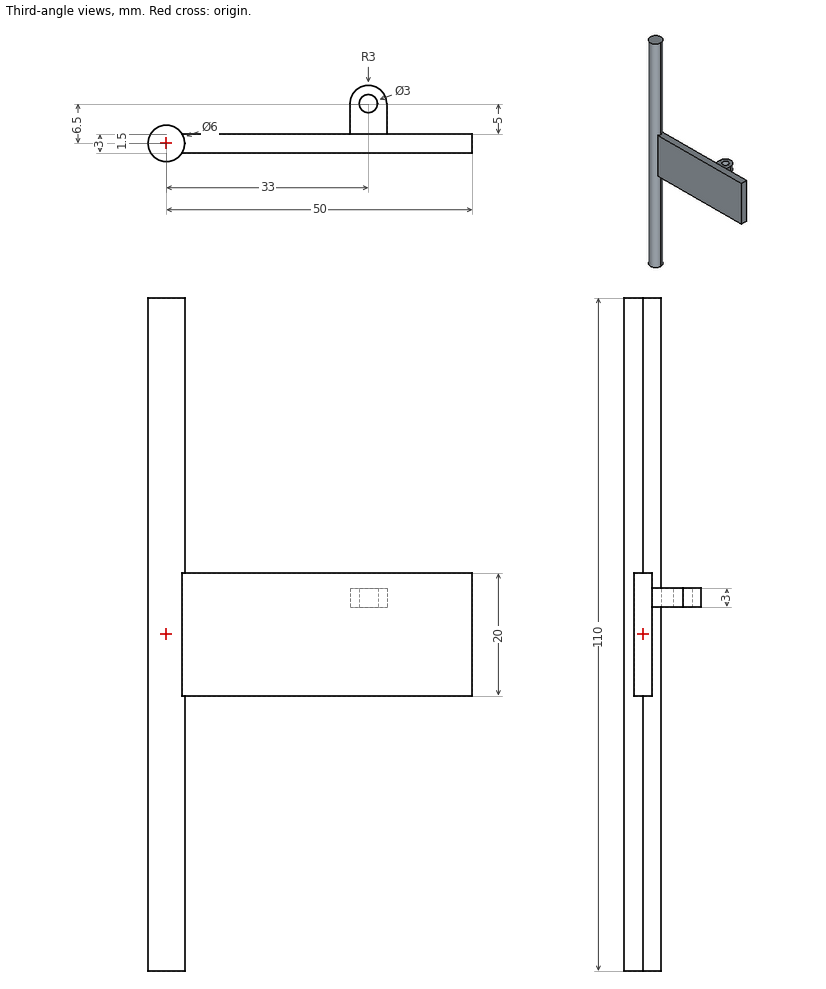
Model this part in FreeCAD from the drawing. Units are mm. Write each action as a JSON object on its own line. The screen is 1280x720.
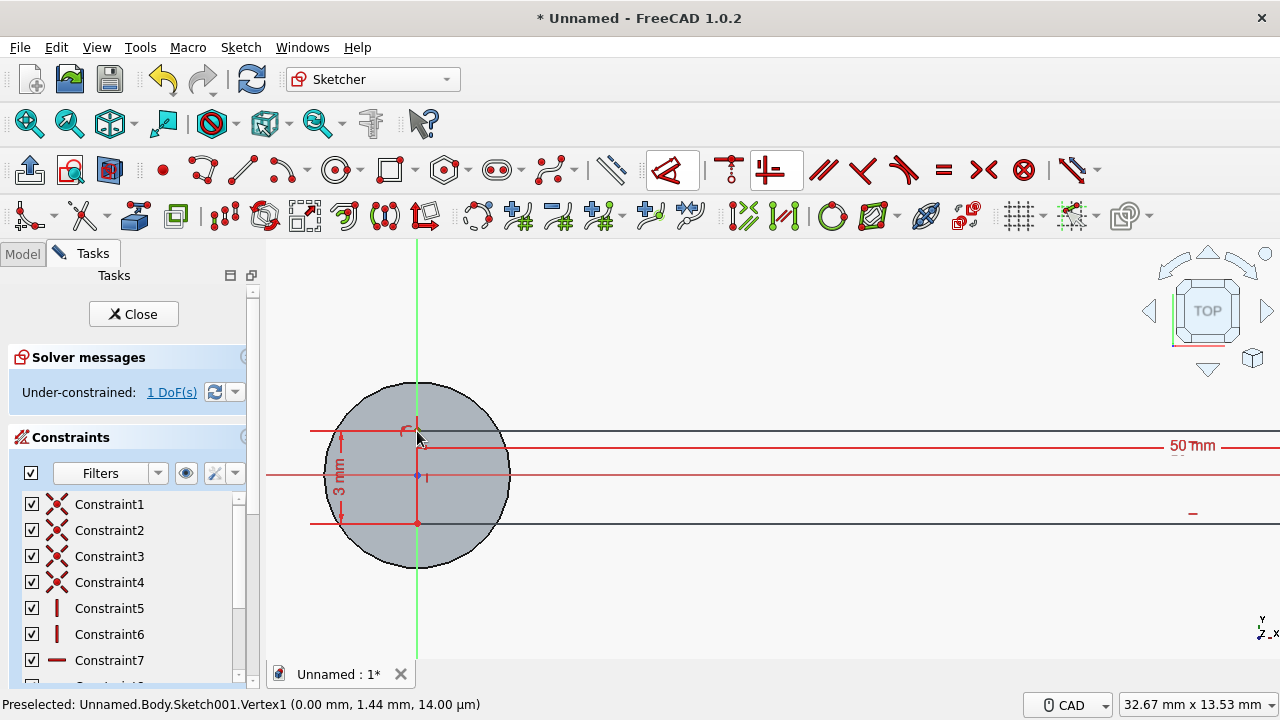
{"action": "key", "text": "i"}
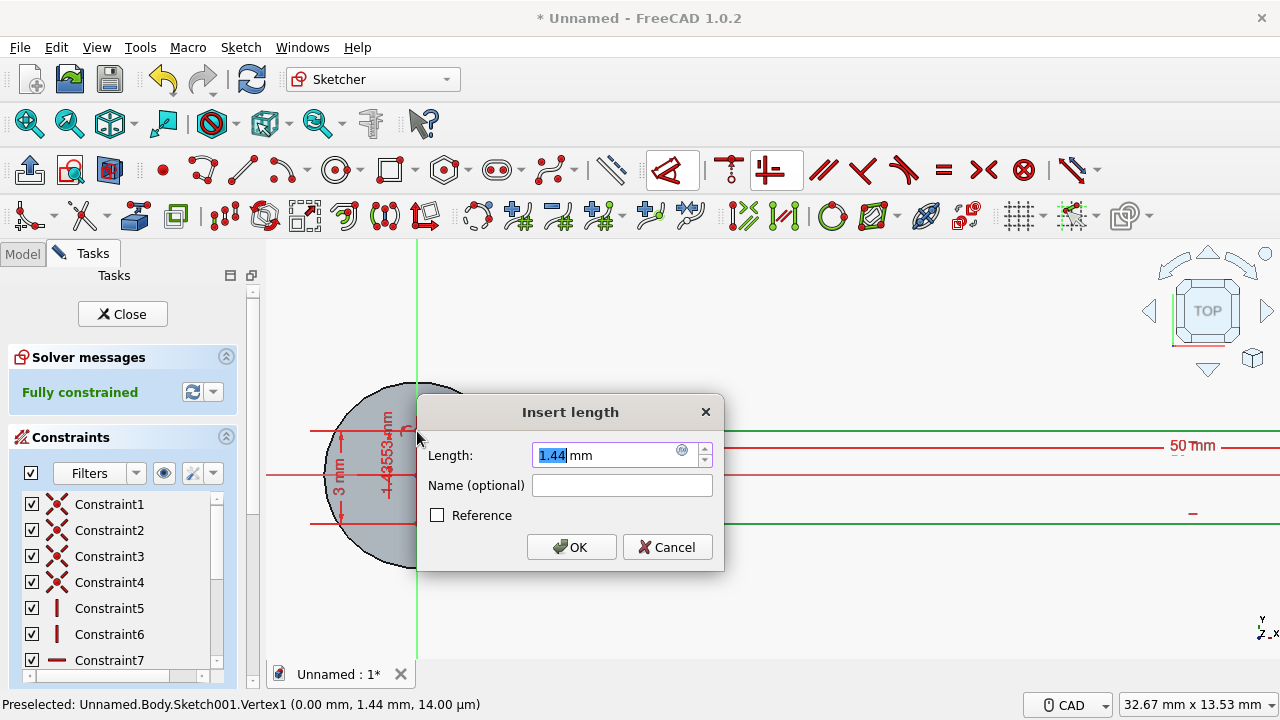
{"action": "type", "text": "1.5"}
{"action": "key", "text": "Return"}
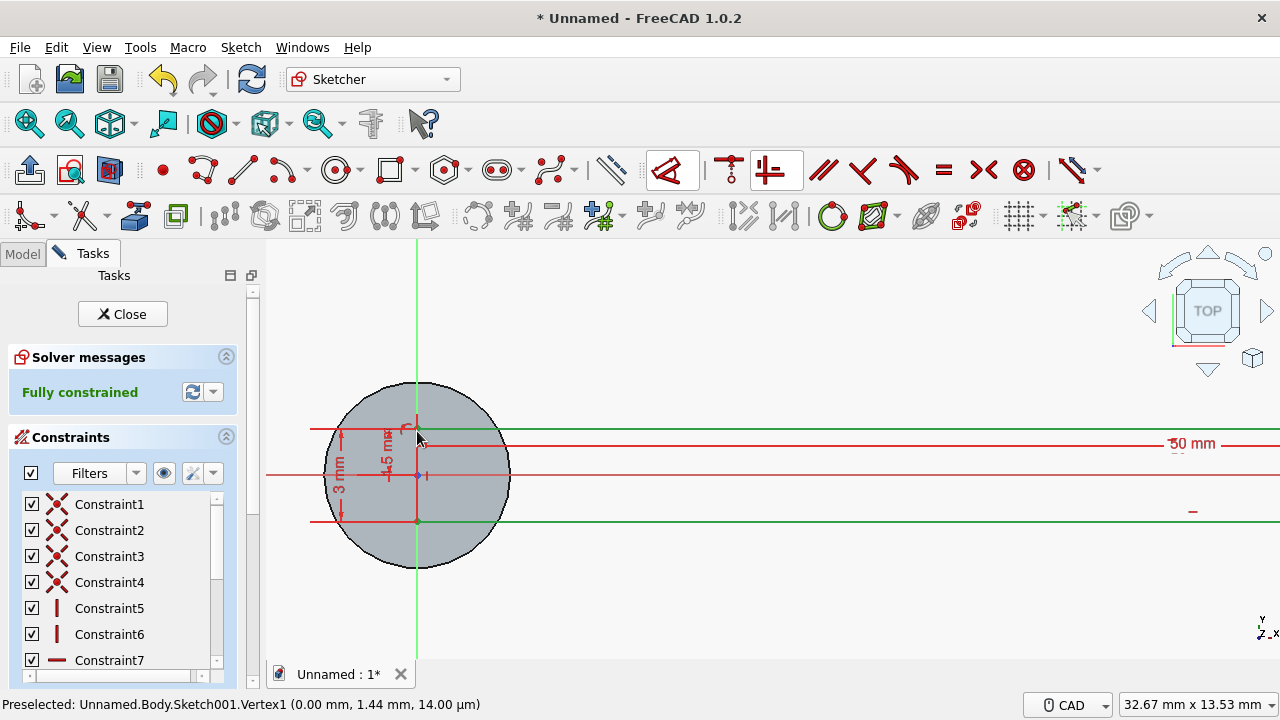
{"action": "left_click", "coordinate": [123, 314]}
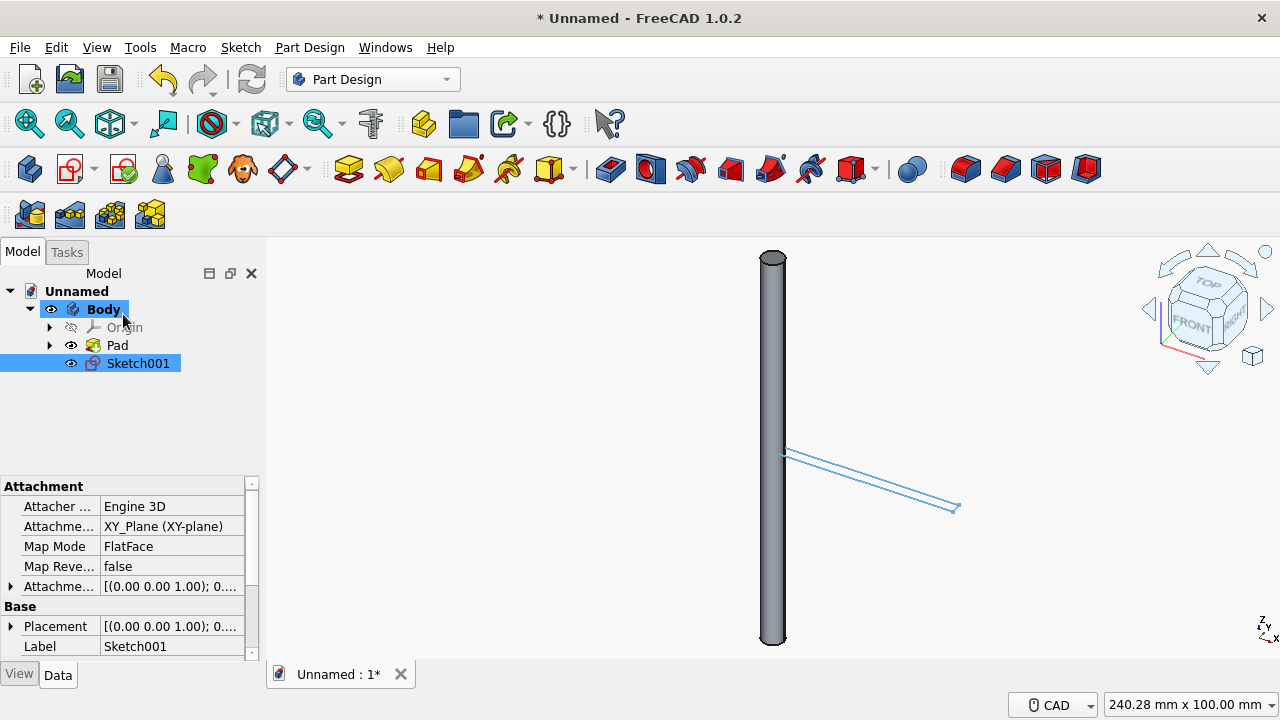
{"action": "left_click", "coordinate": [350, 170]}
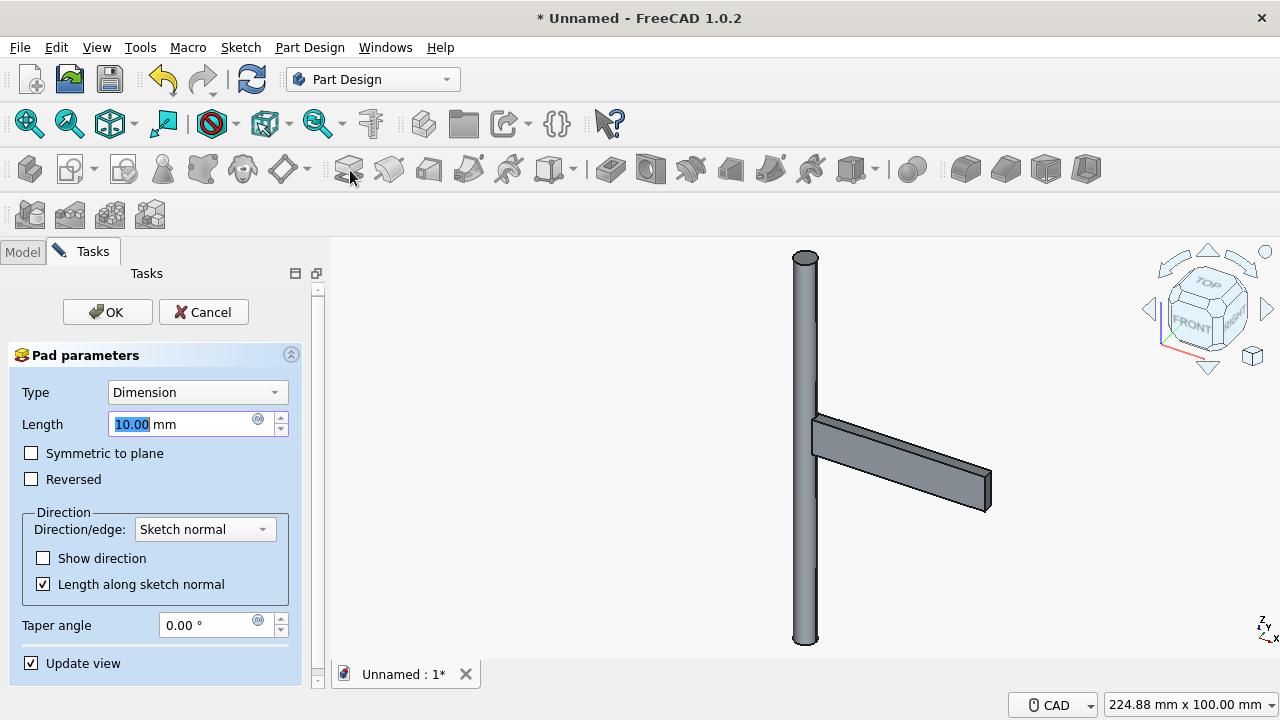
{"action": "type", "text": "20"}
{"action": "key", "text": "Tab"}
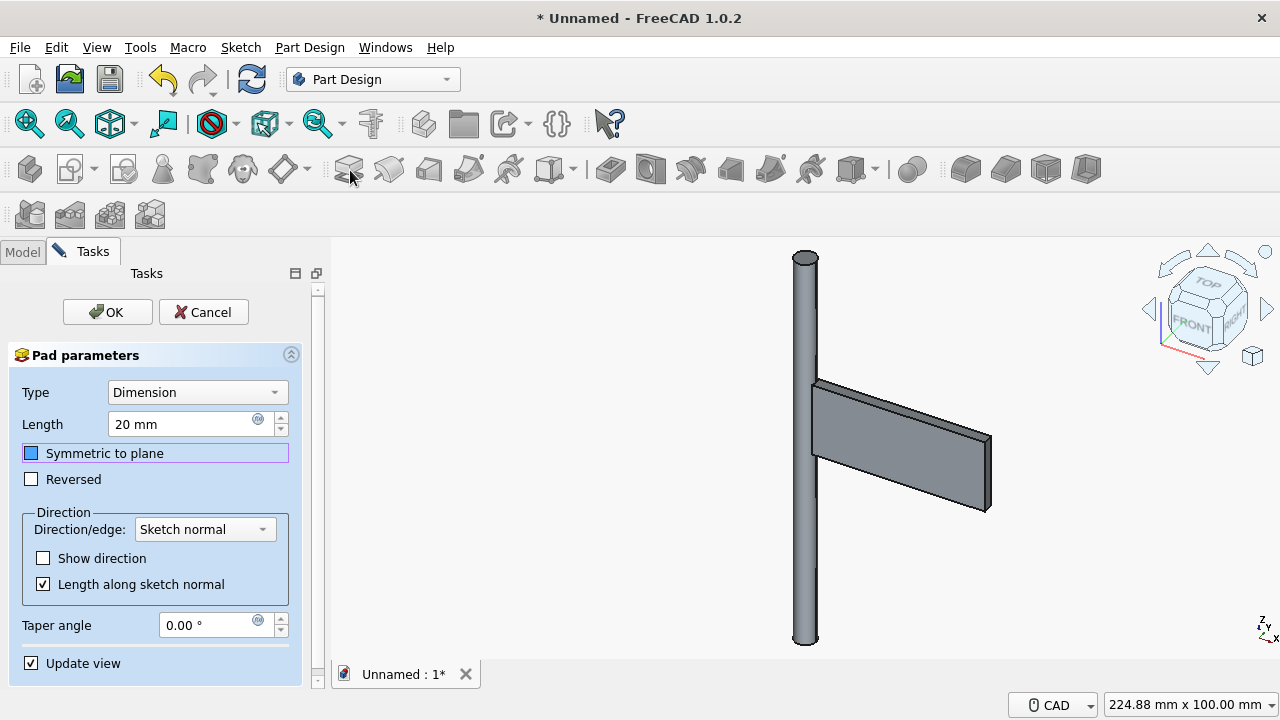
{"action": "left_click", "coordinate": [30, 453]}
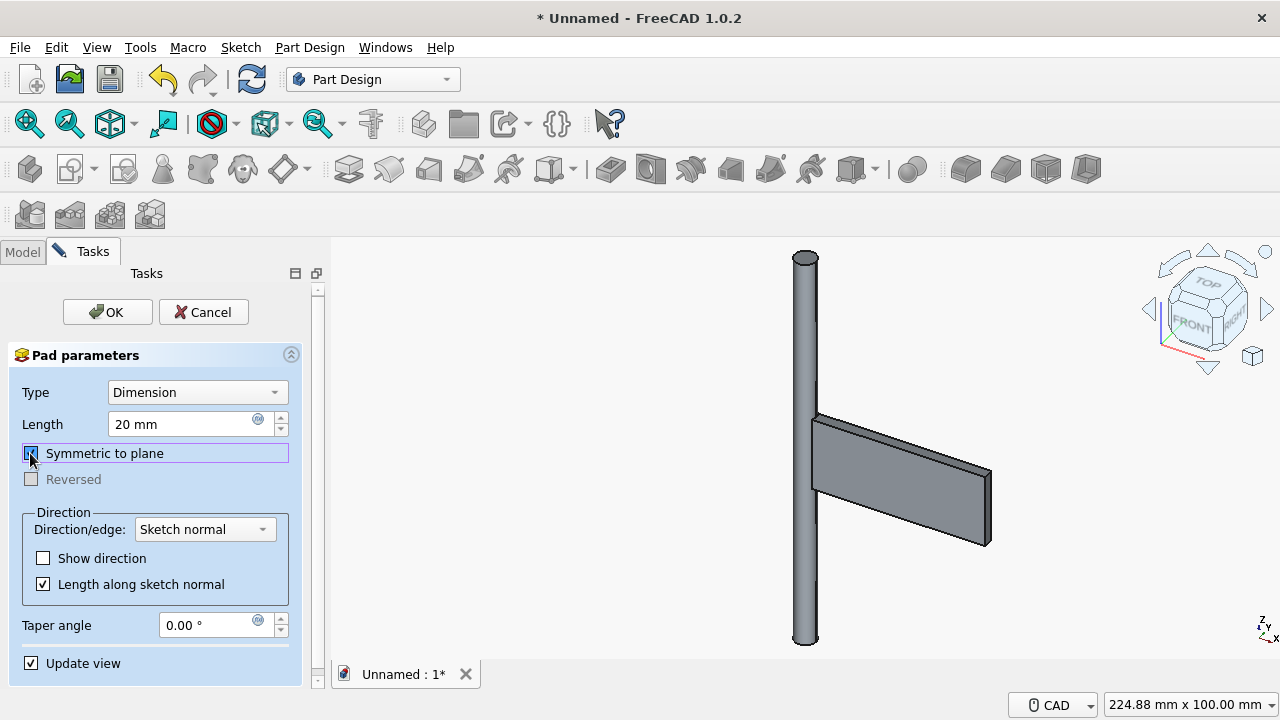
{"action": "left_click", "coordinate": [108, 312]}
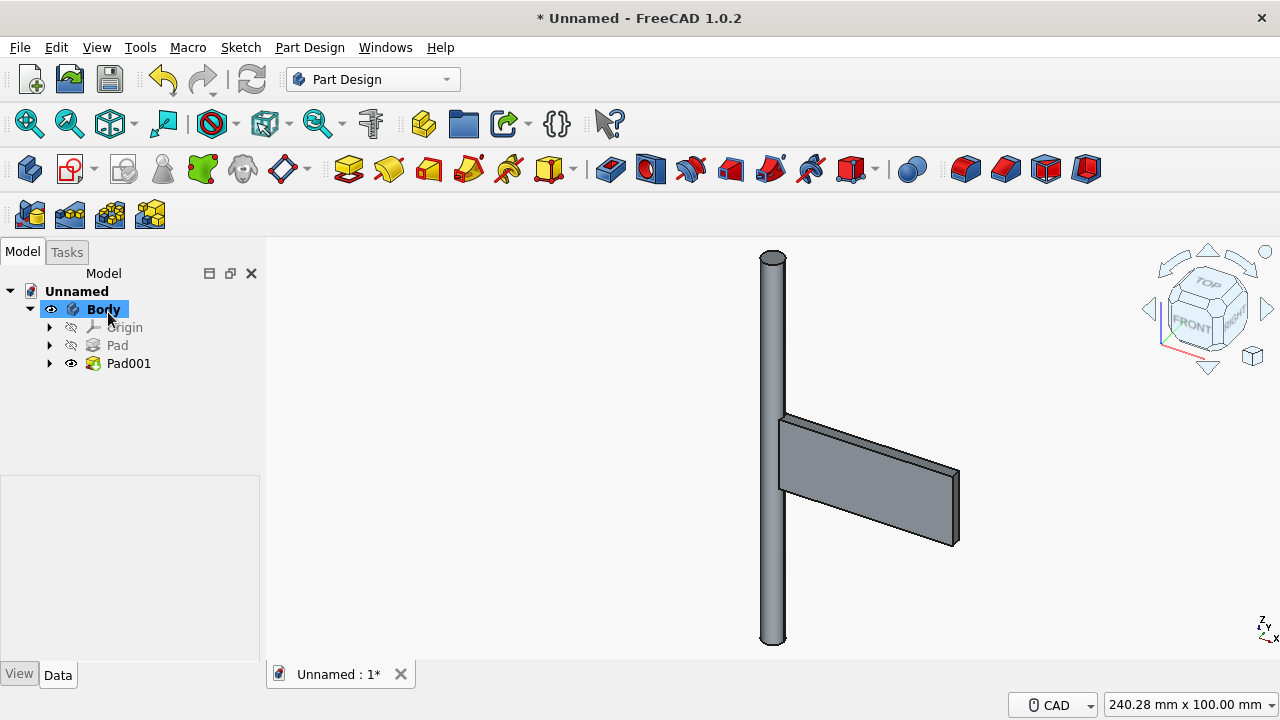
{"action": "left_click", "coordinate": [30, 124]}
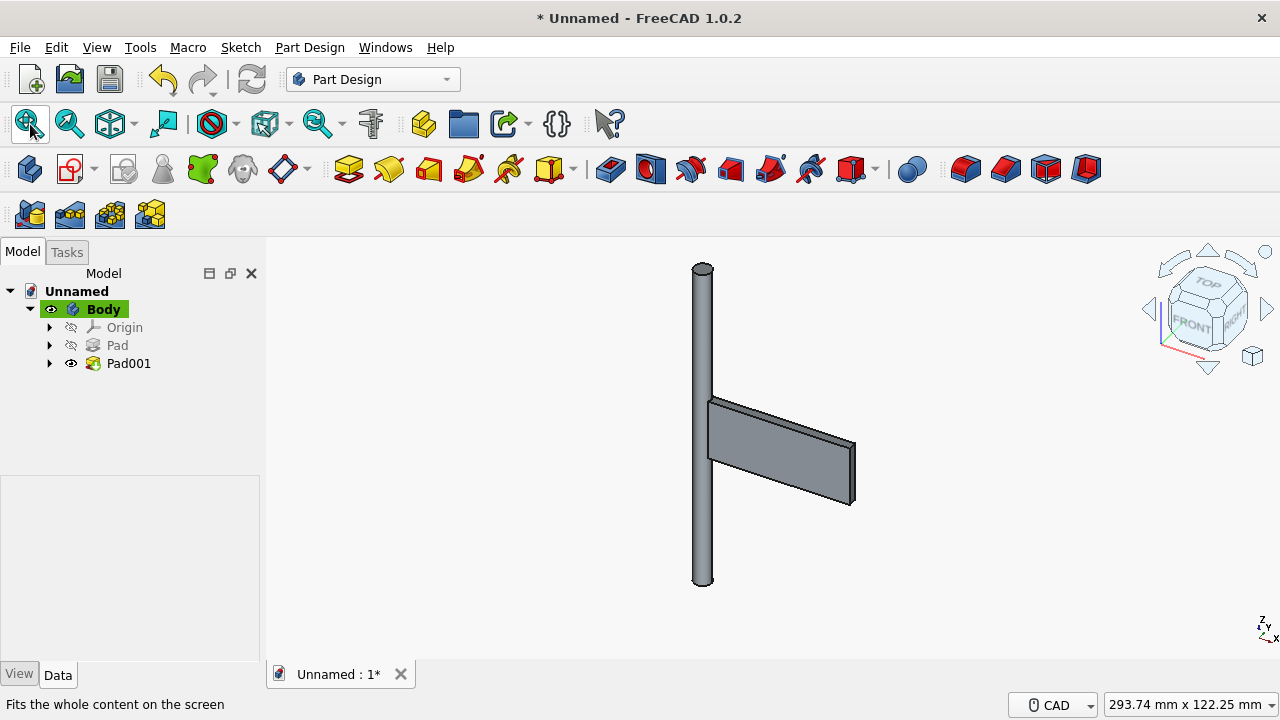
{"action": "left_click", "coordinate": [50, 327]}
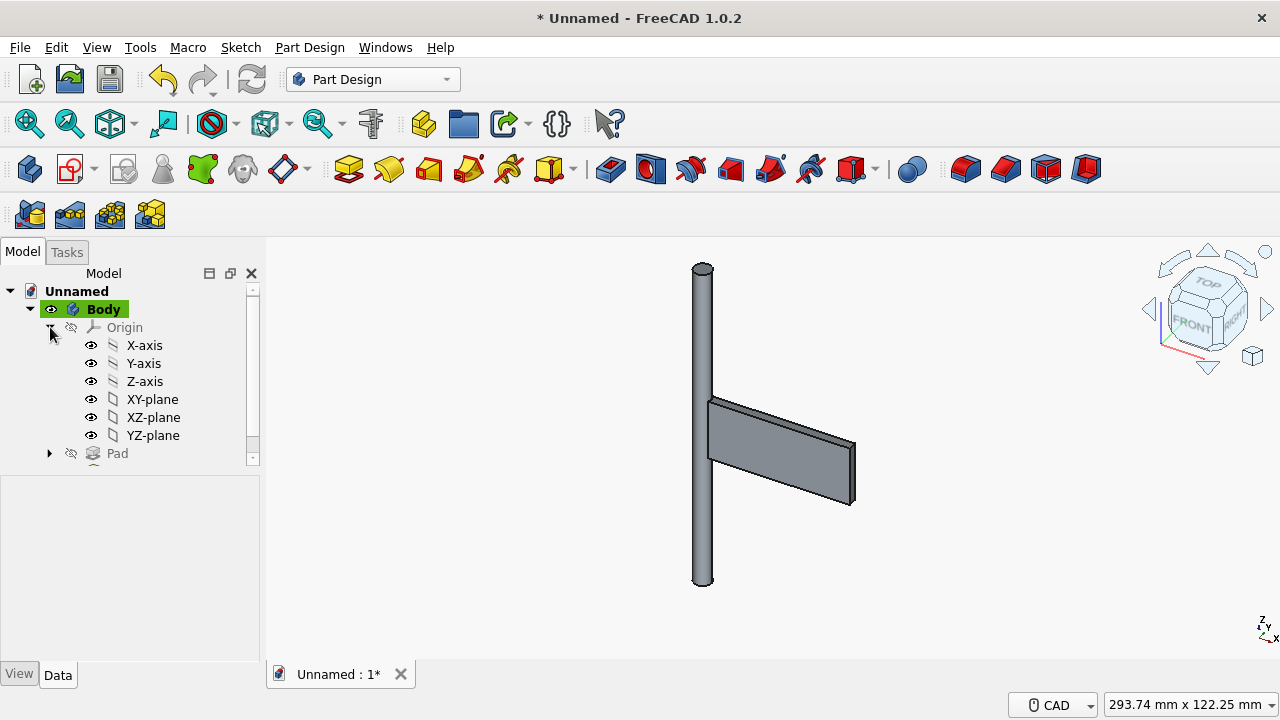
{"action": "left_click", "coordinate": [136, 399]}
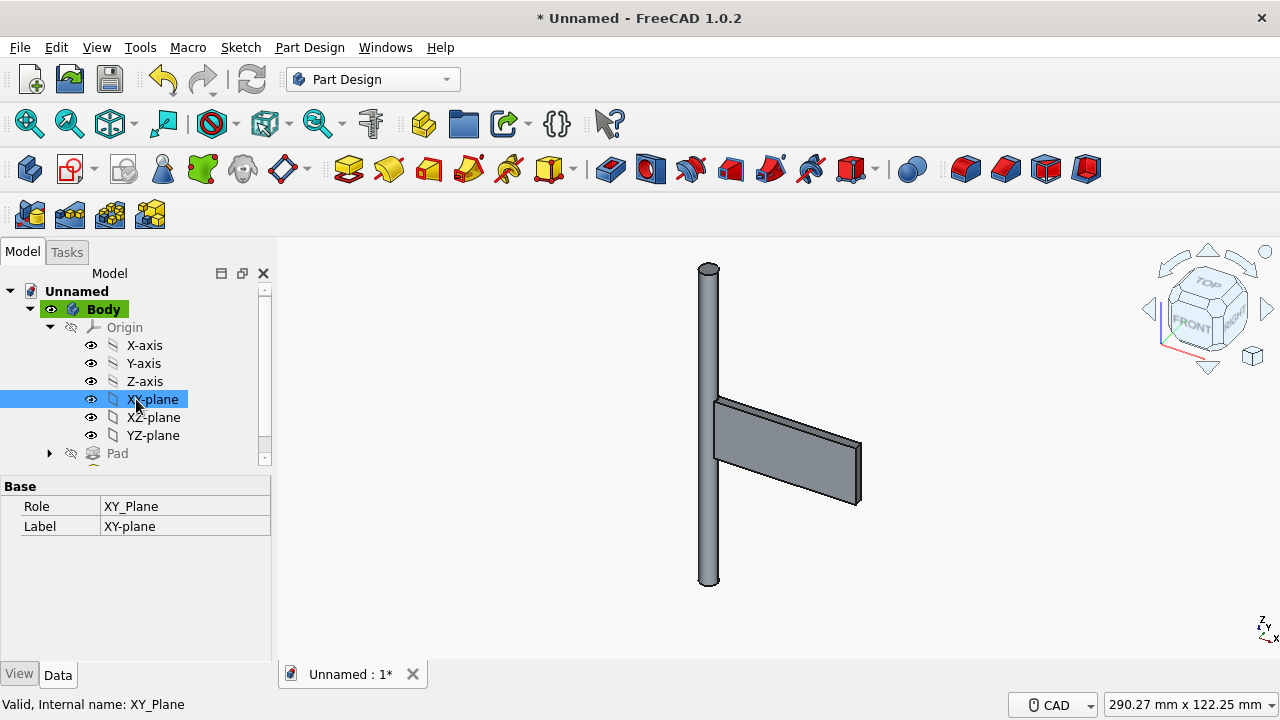
{"action": "left_click", "coordinate": [284, 170]}